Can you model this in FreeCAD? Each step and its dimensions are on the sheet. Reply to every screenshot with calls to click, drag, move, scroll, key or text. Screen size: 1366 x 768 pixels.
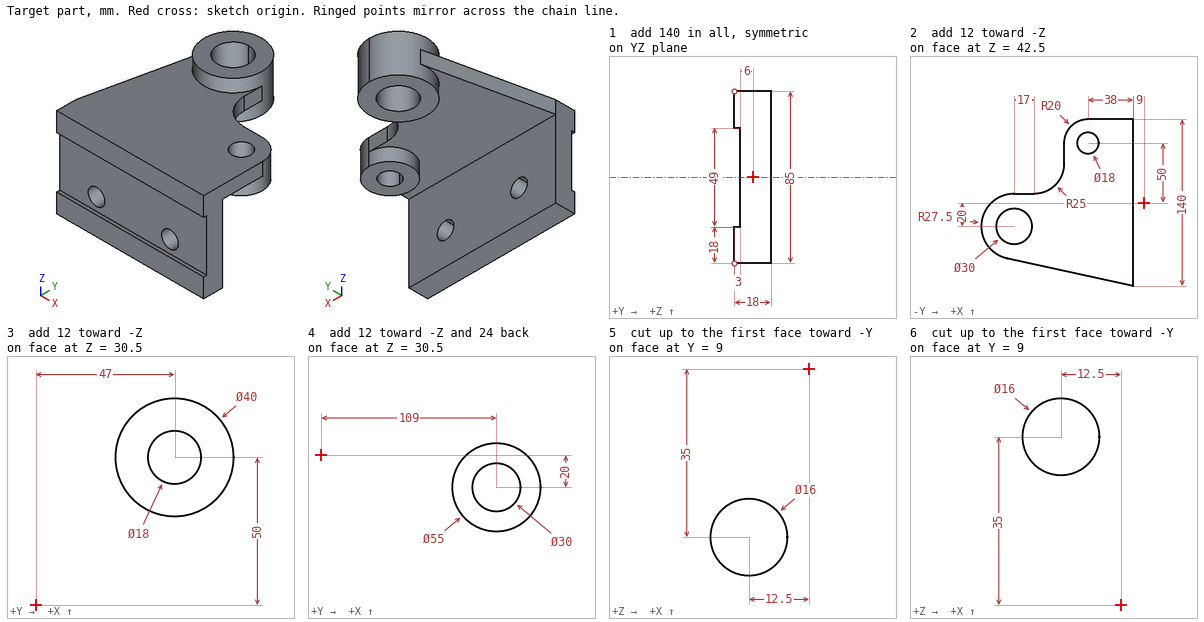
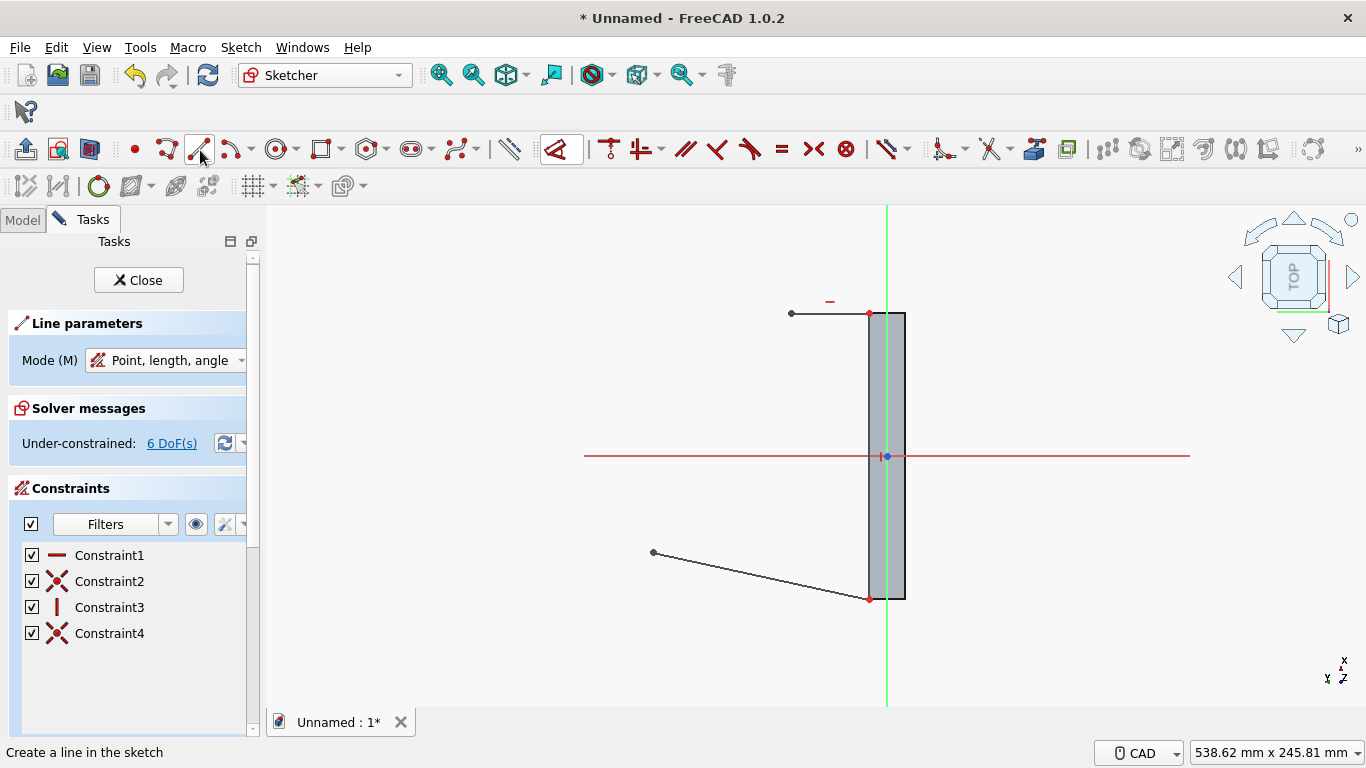
click(665, 441)
click(699, 441)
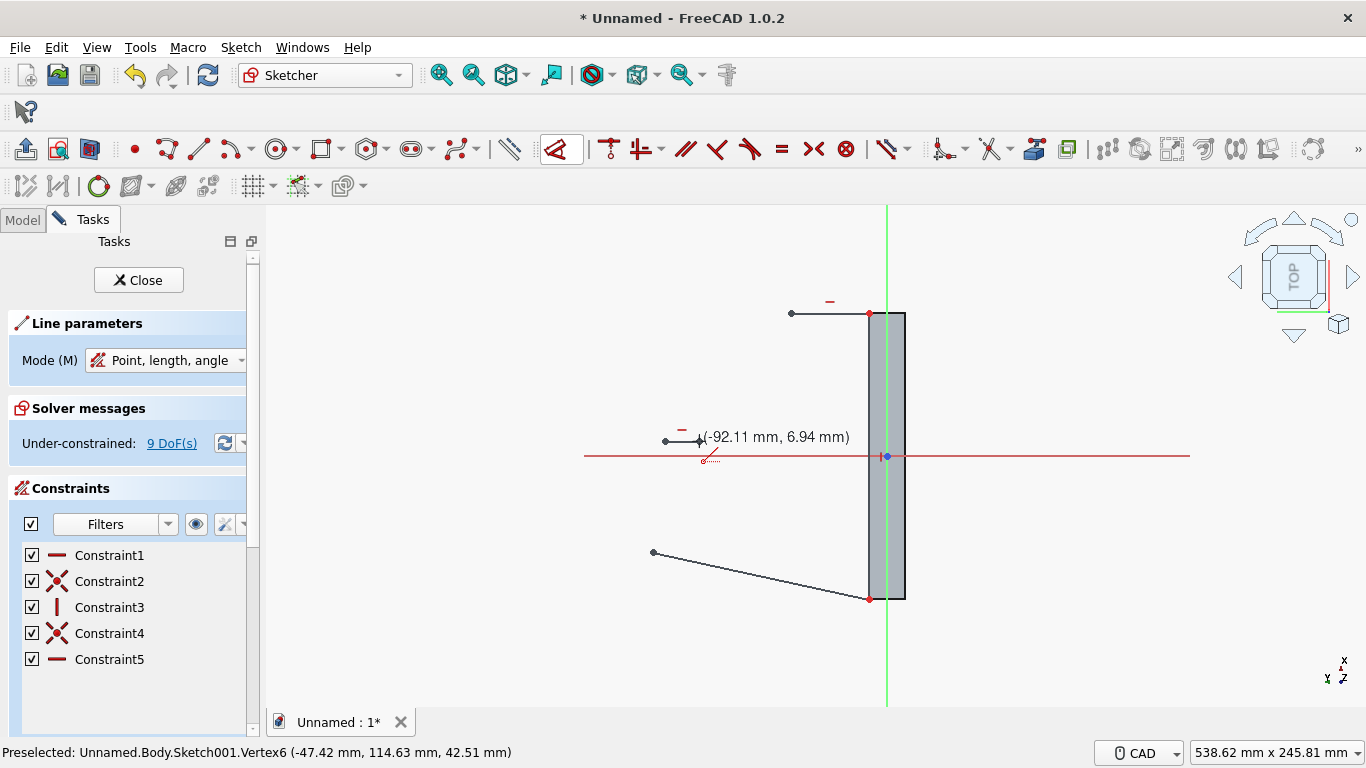
click(750, 390)
click(750, 354)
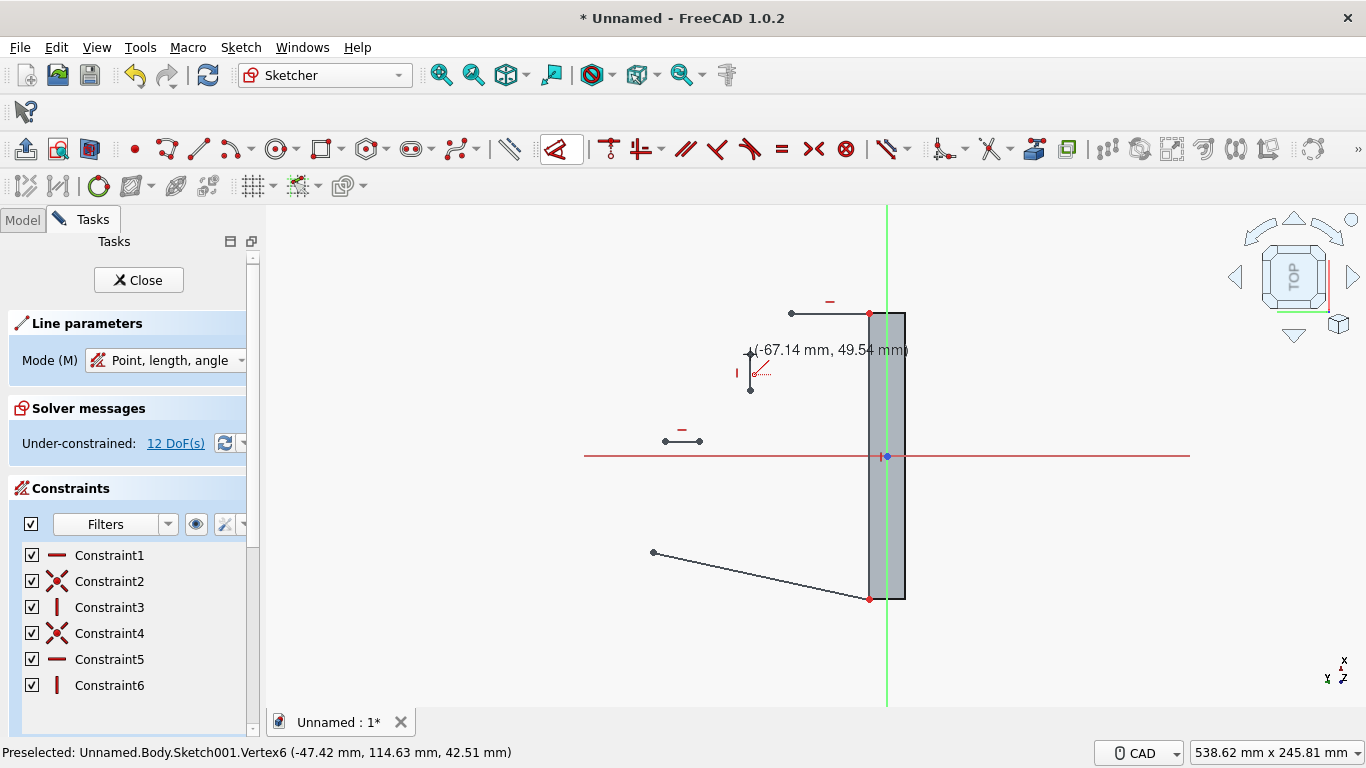
key(g)
key(3)
key(a)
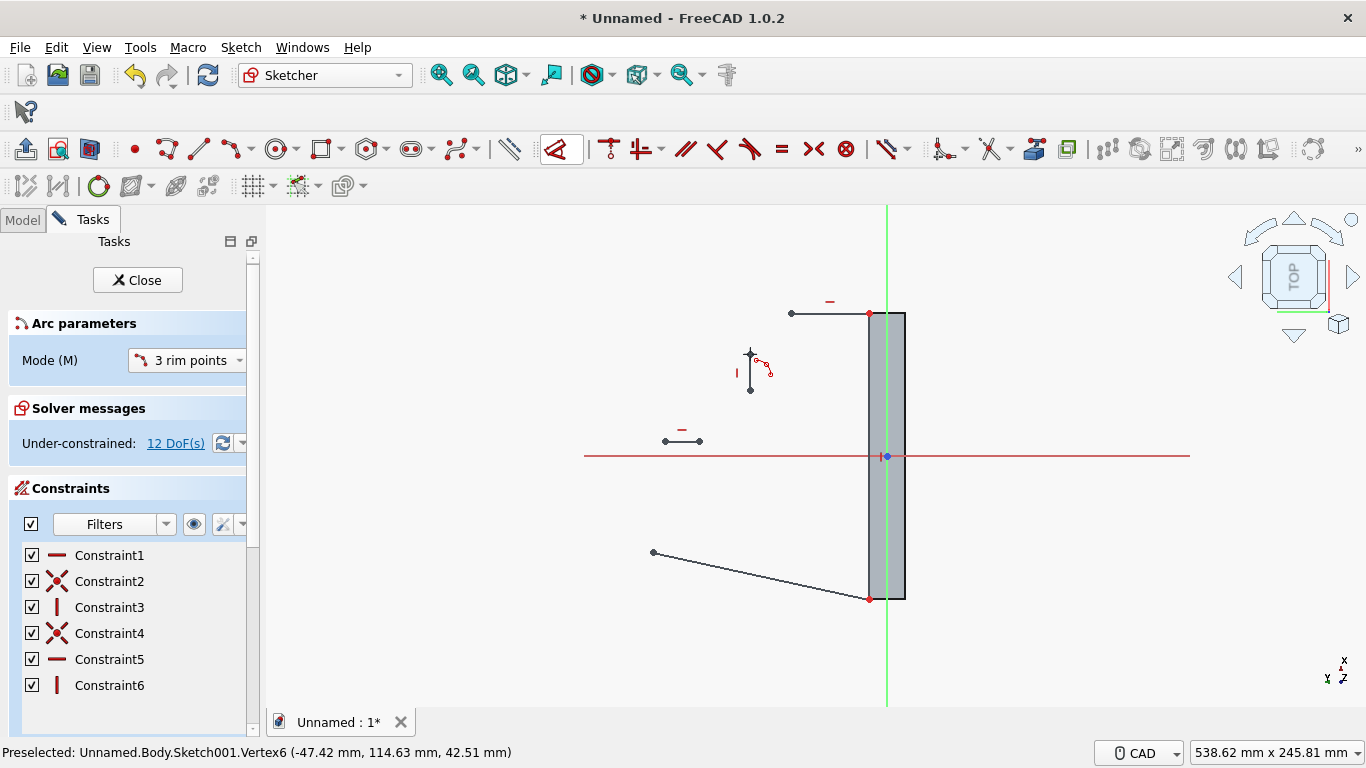
click(653, 553)
click(665, 442)
click(609, 491)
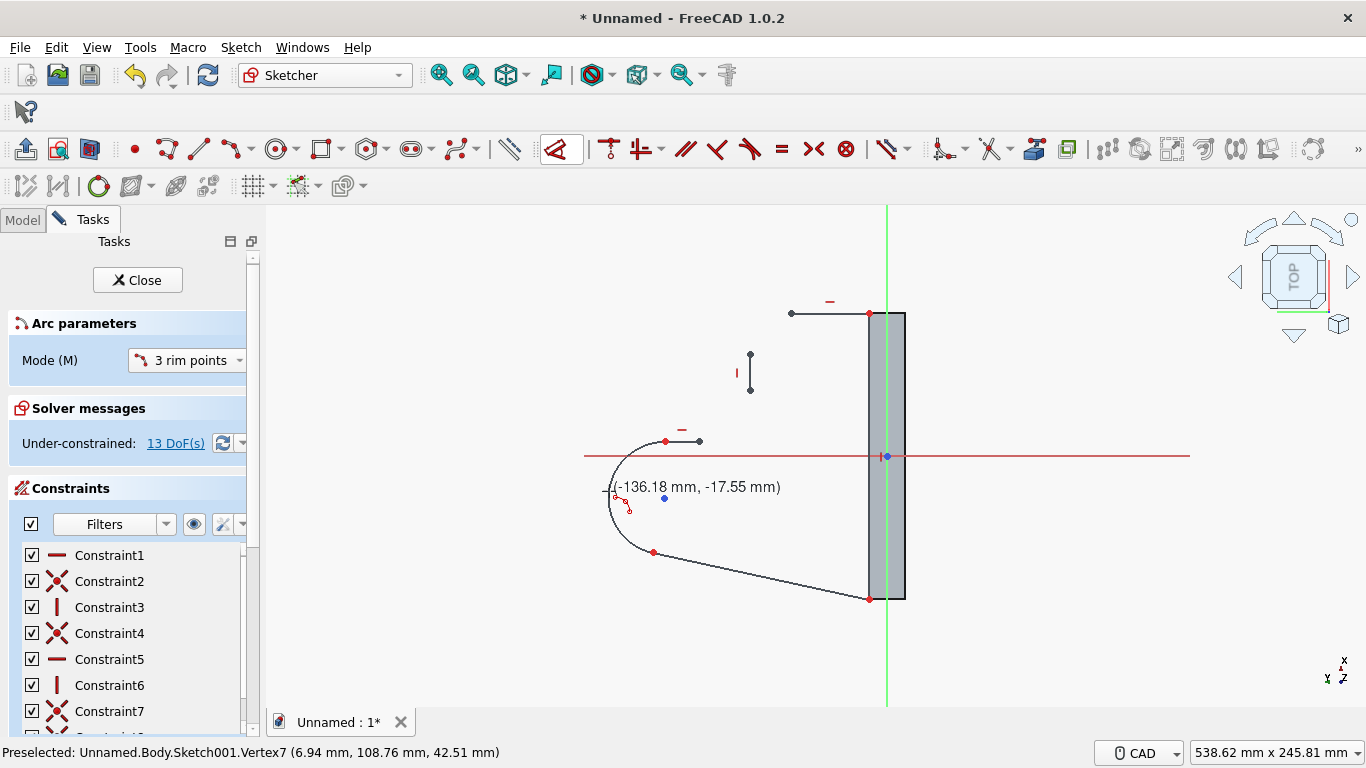
click(699, 442)
click(750, 391)
click(735, 426)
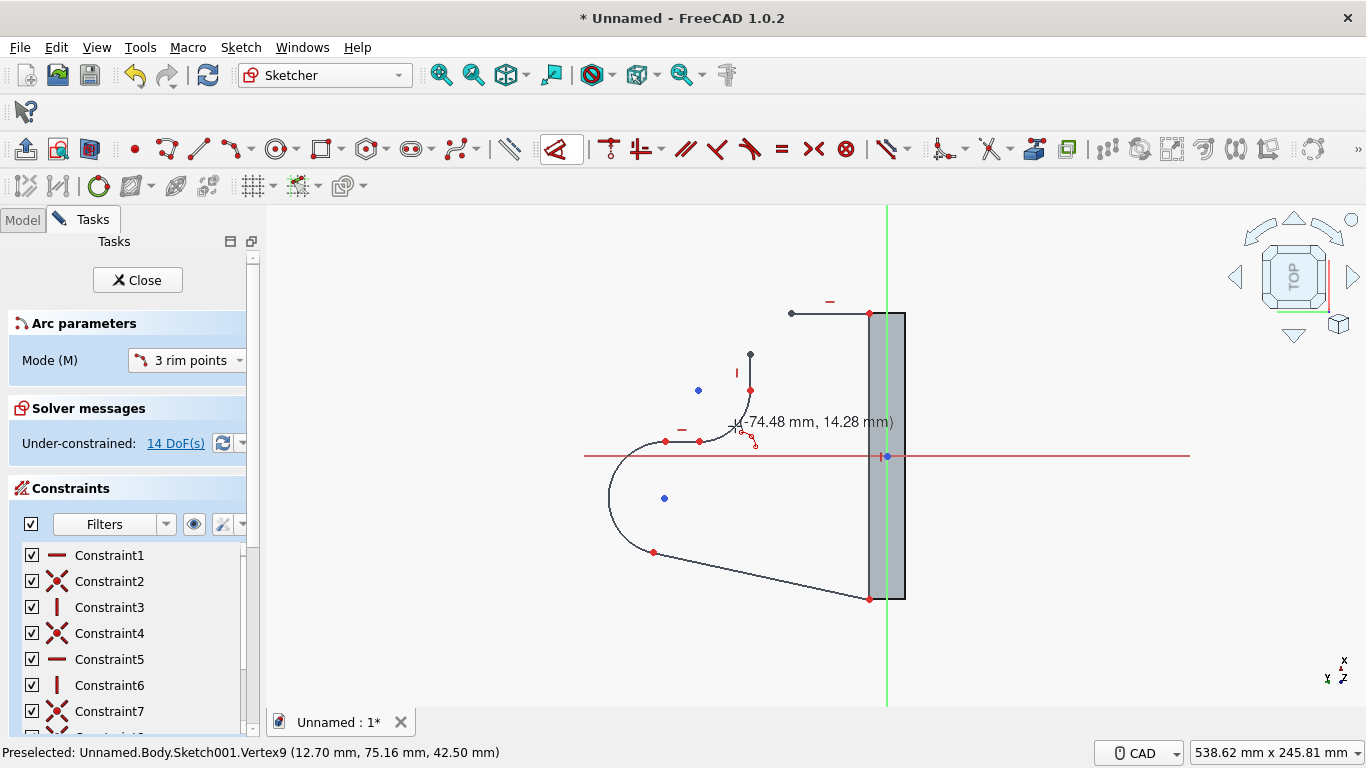
click(750, 355)
click(791, 314)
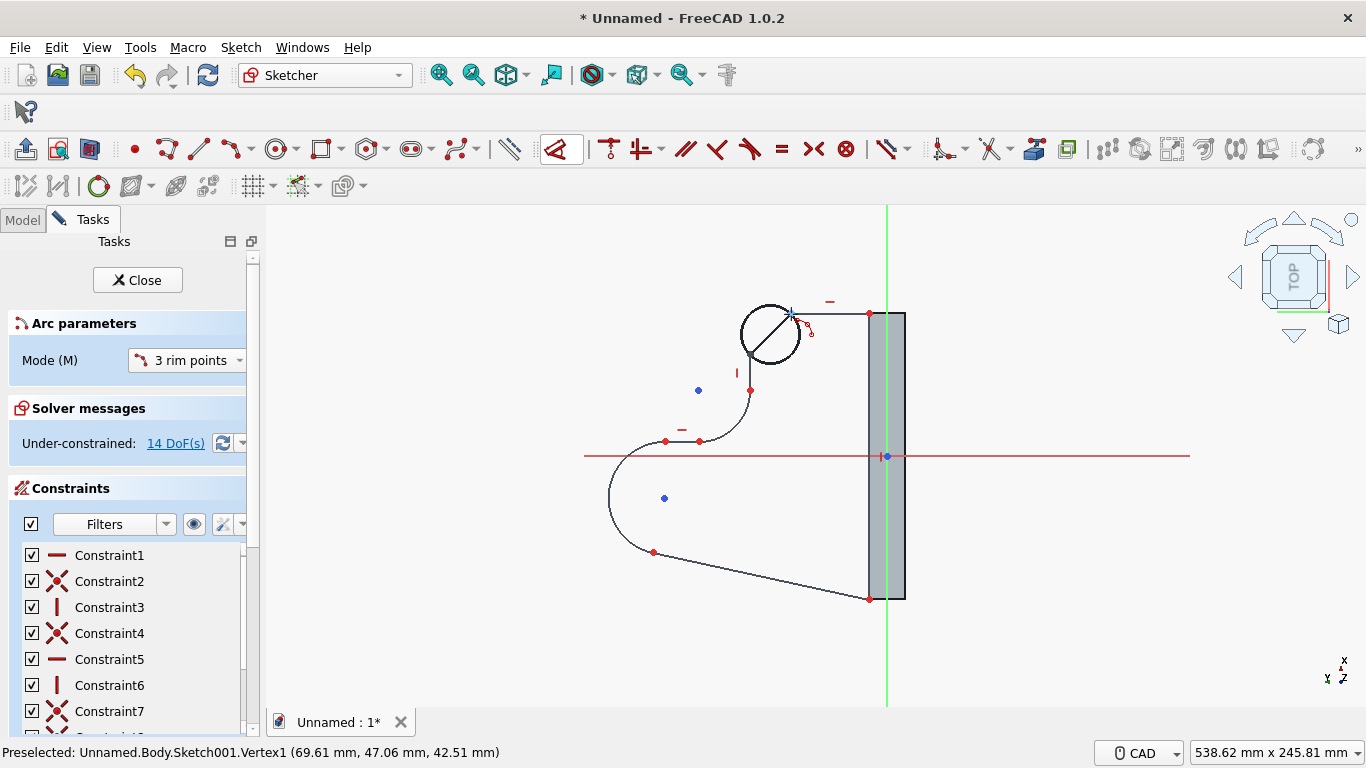
scroll(762, 325, up, 2)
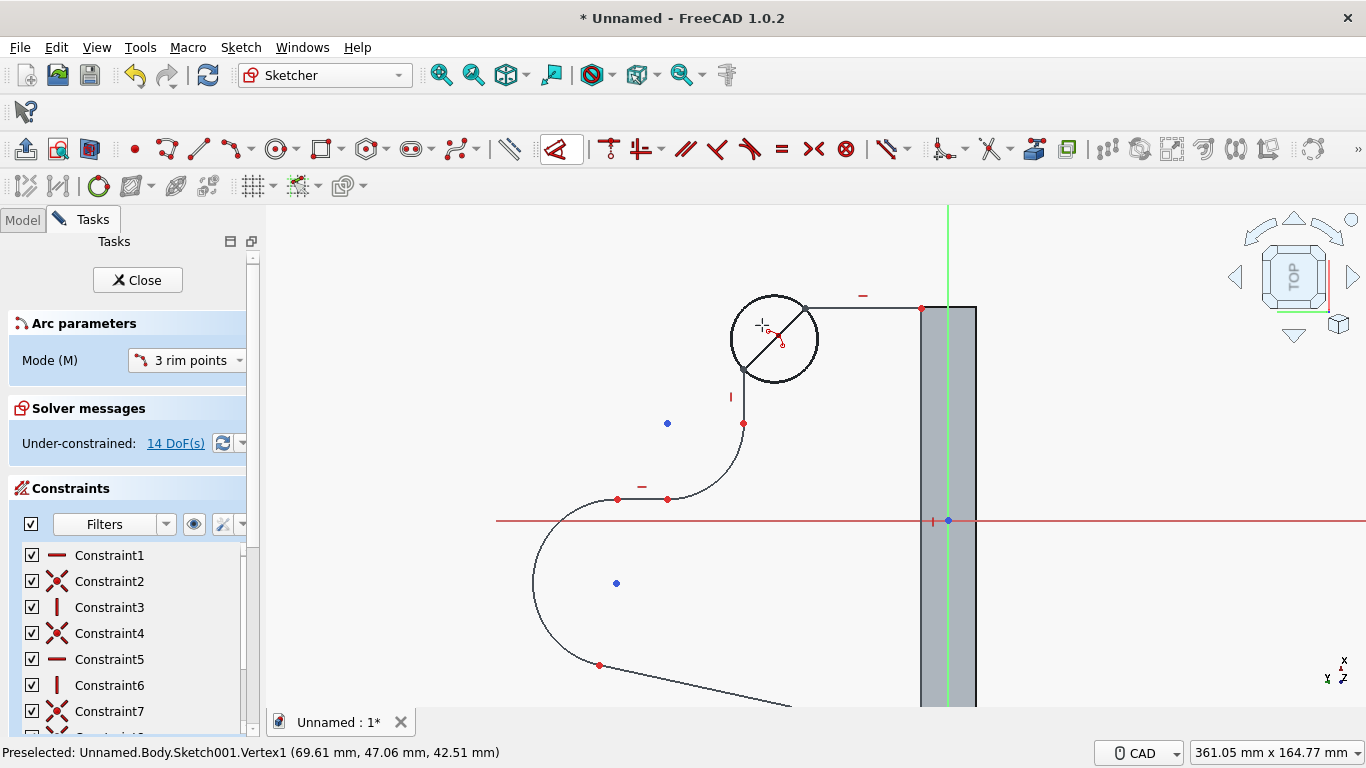
click(762, 325)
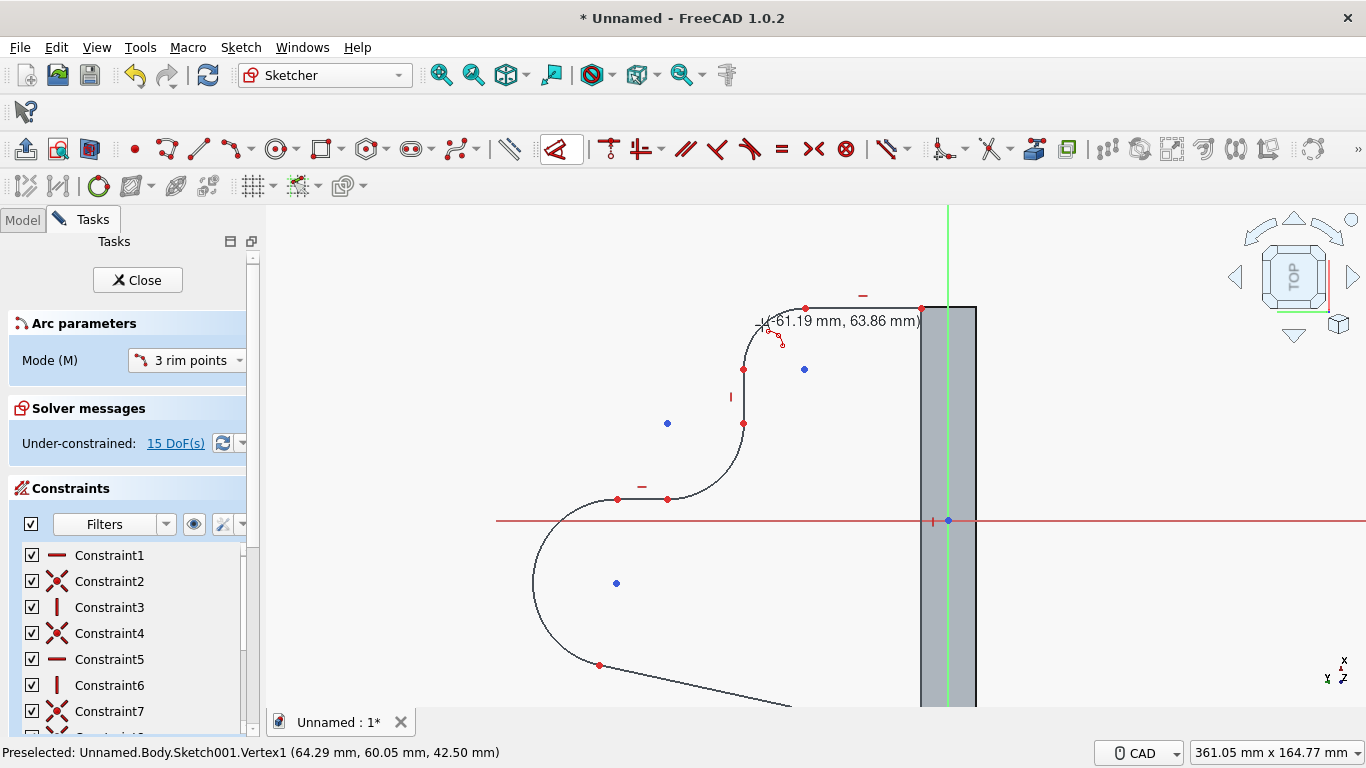
key(g)
key(c)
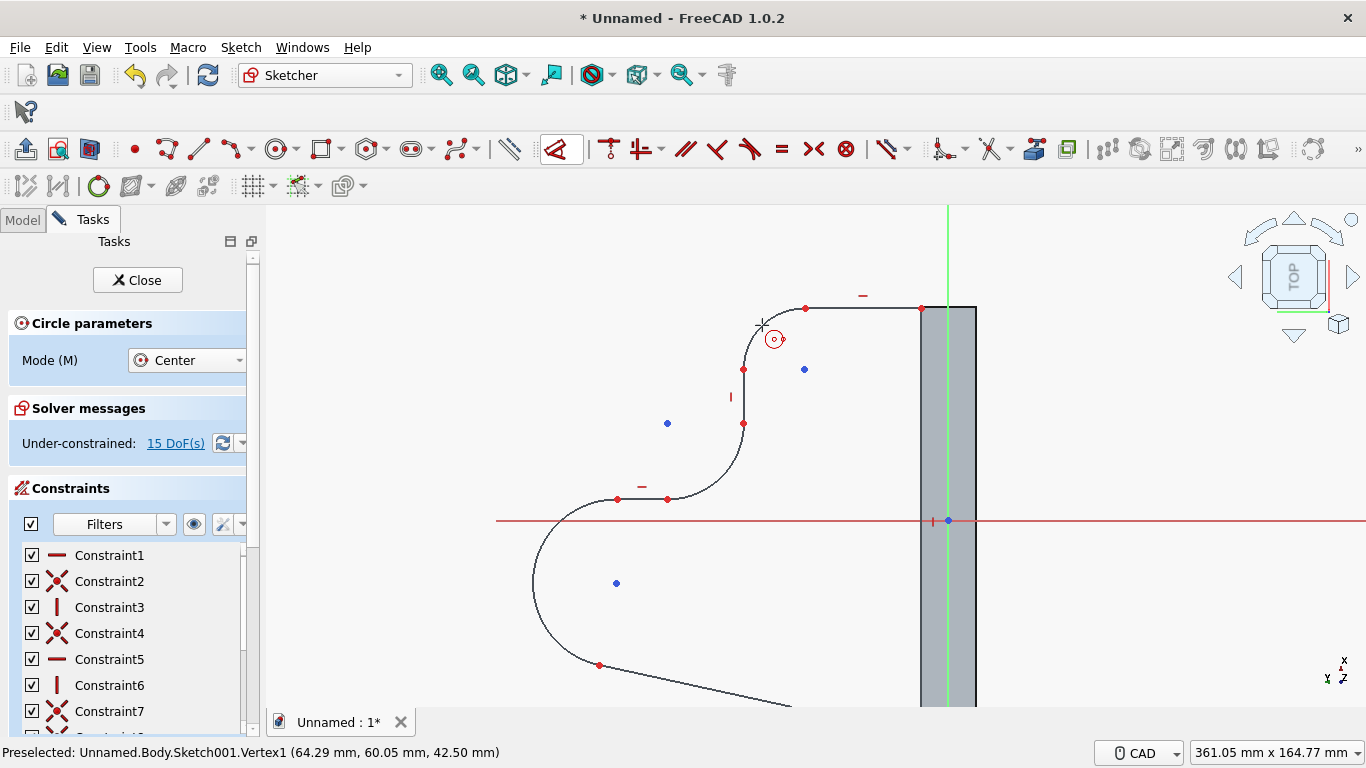
click(805, 368)
move(825, 349)